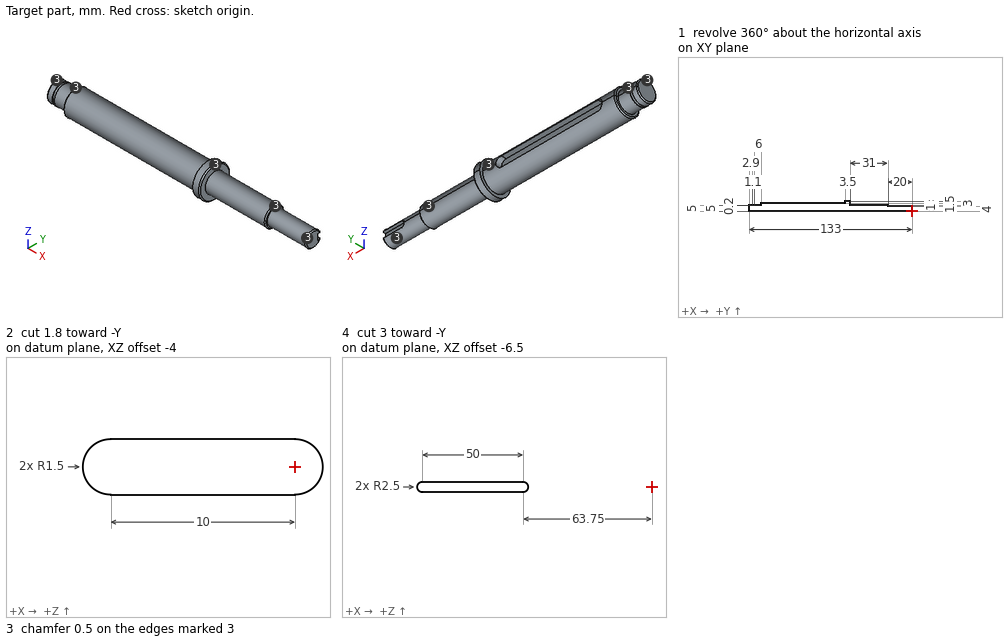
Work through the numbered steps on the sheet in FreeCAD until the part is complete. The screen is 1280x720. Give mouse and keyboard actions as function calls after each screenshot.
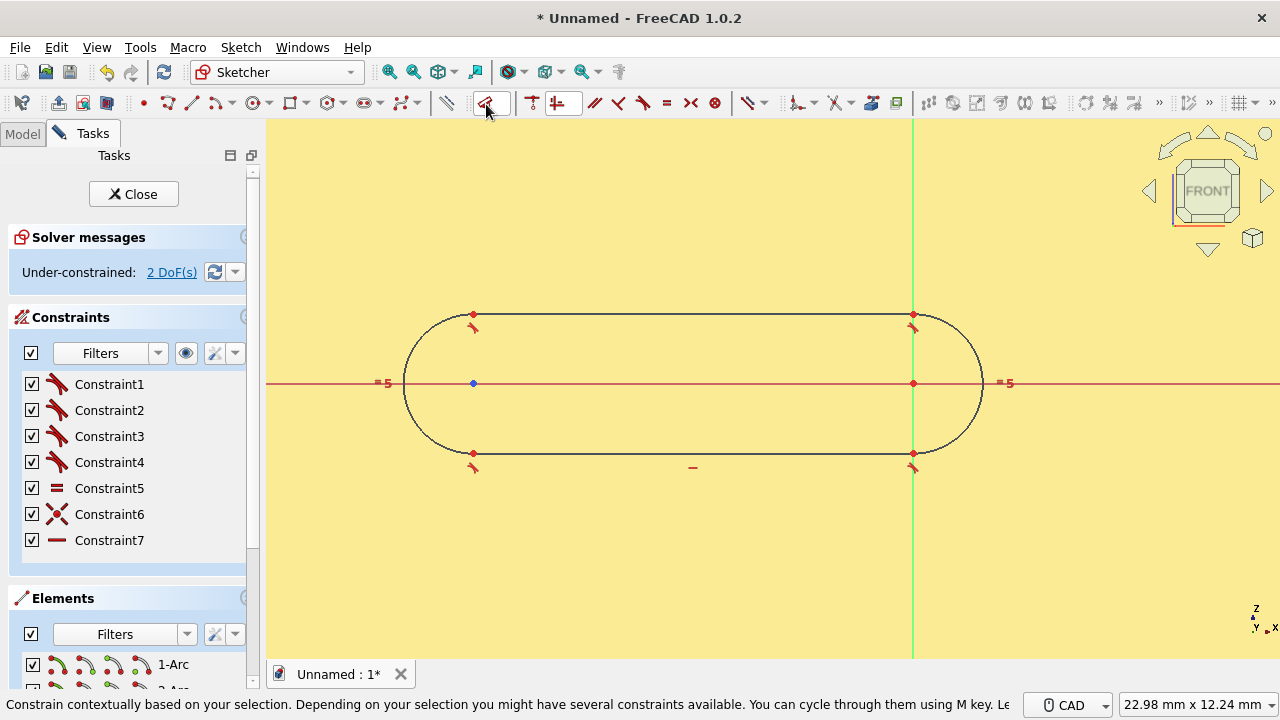
click(970, 425)
click(996, 444)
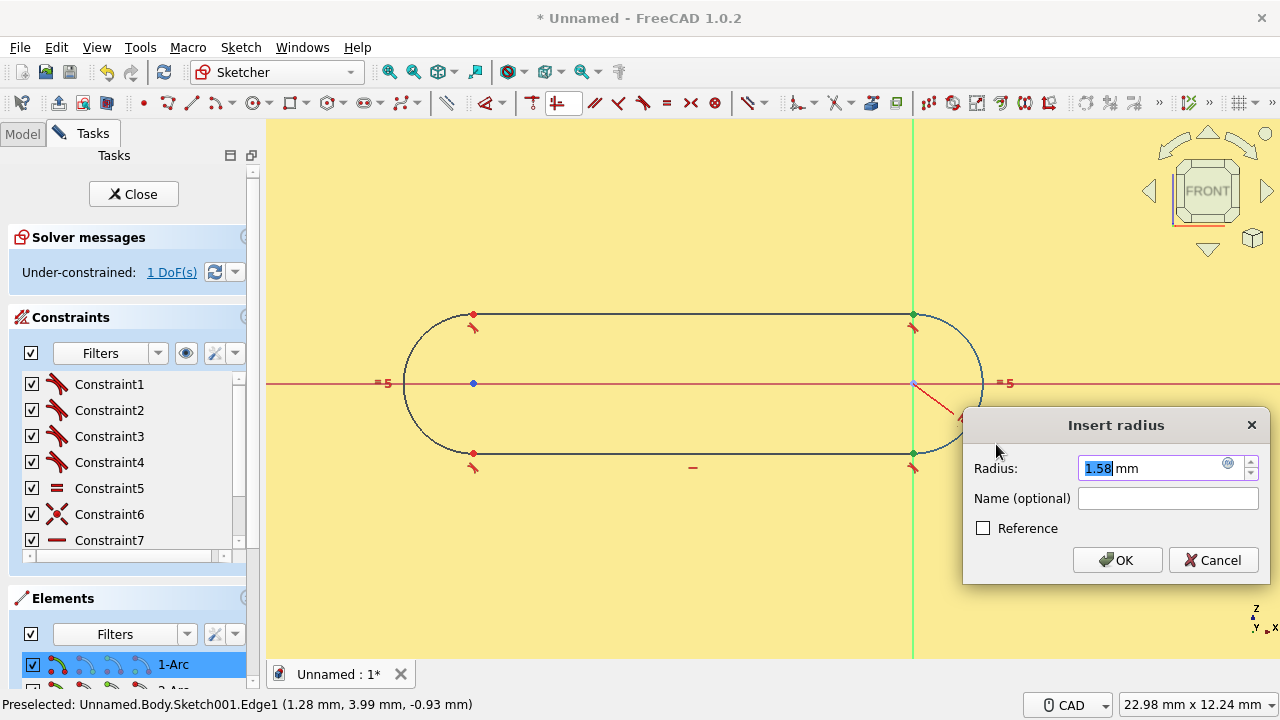
text(1.5)
key(Return)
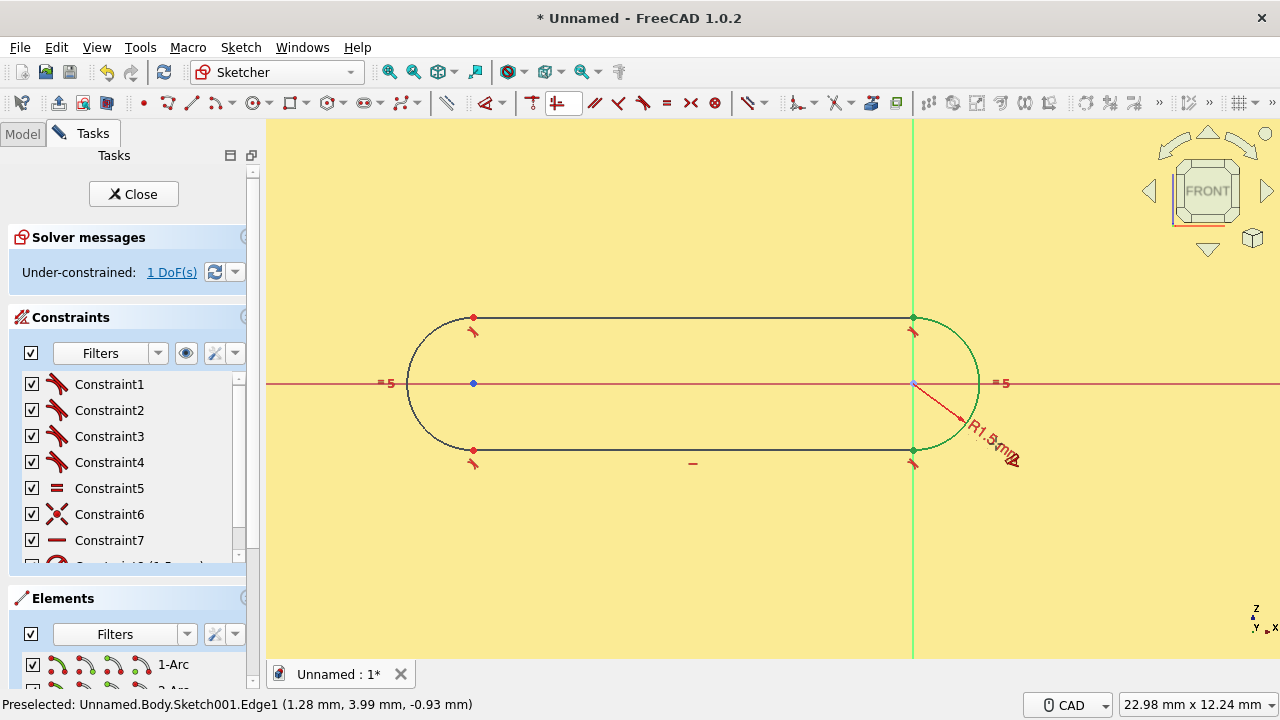
click(781, 450)
click(693, 484)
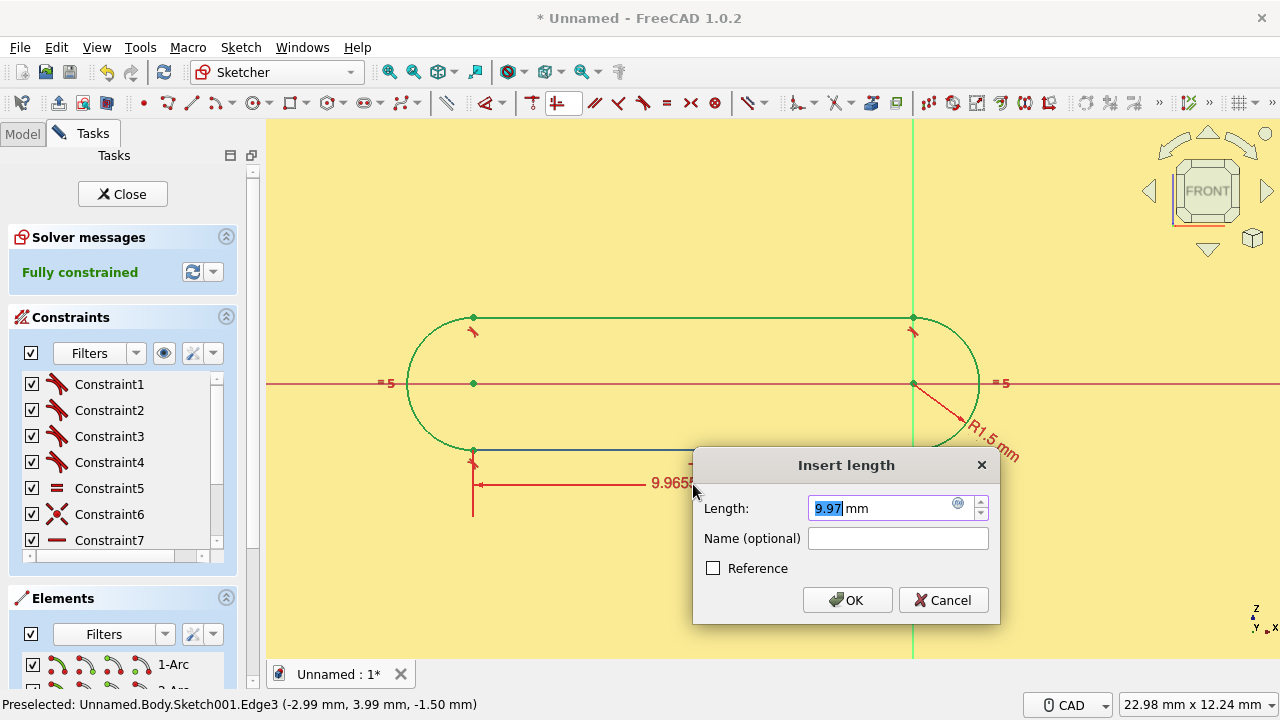
text(10)
key(Return)
key(Escape)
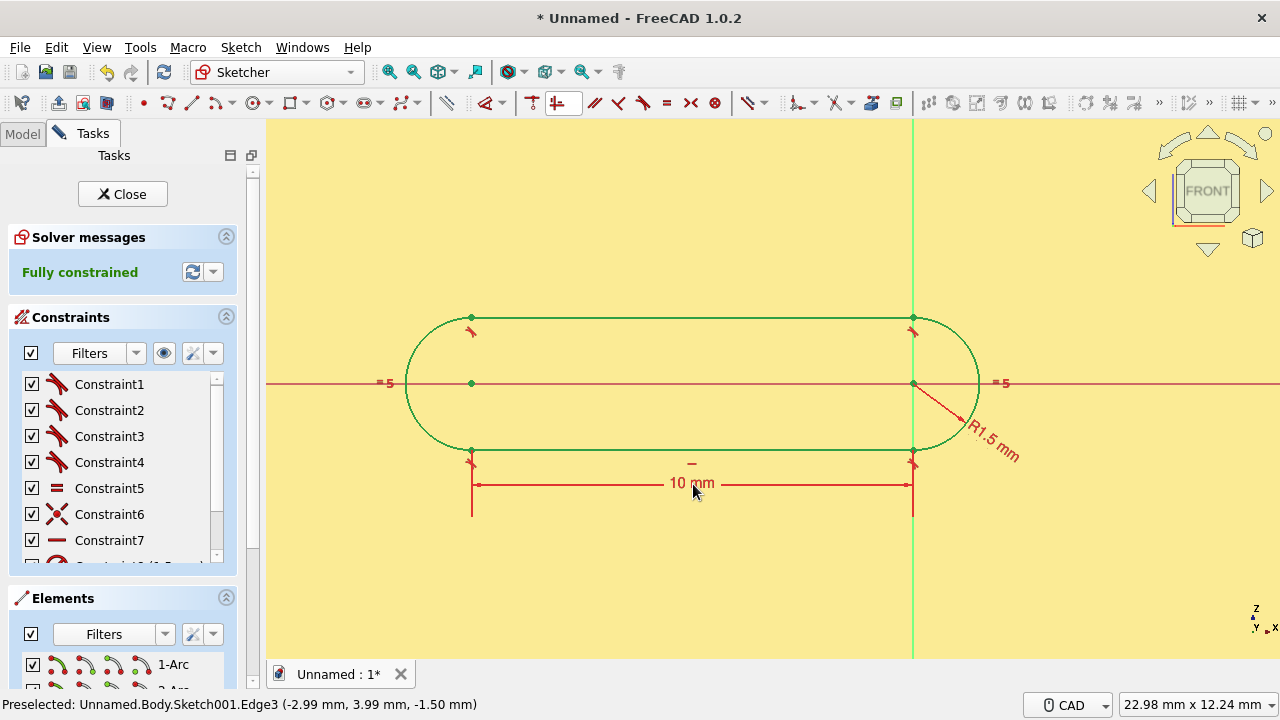
click(123, 194)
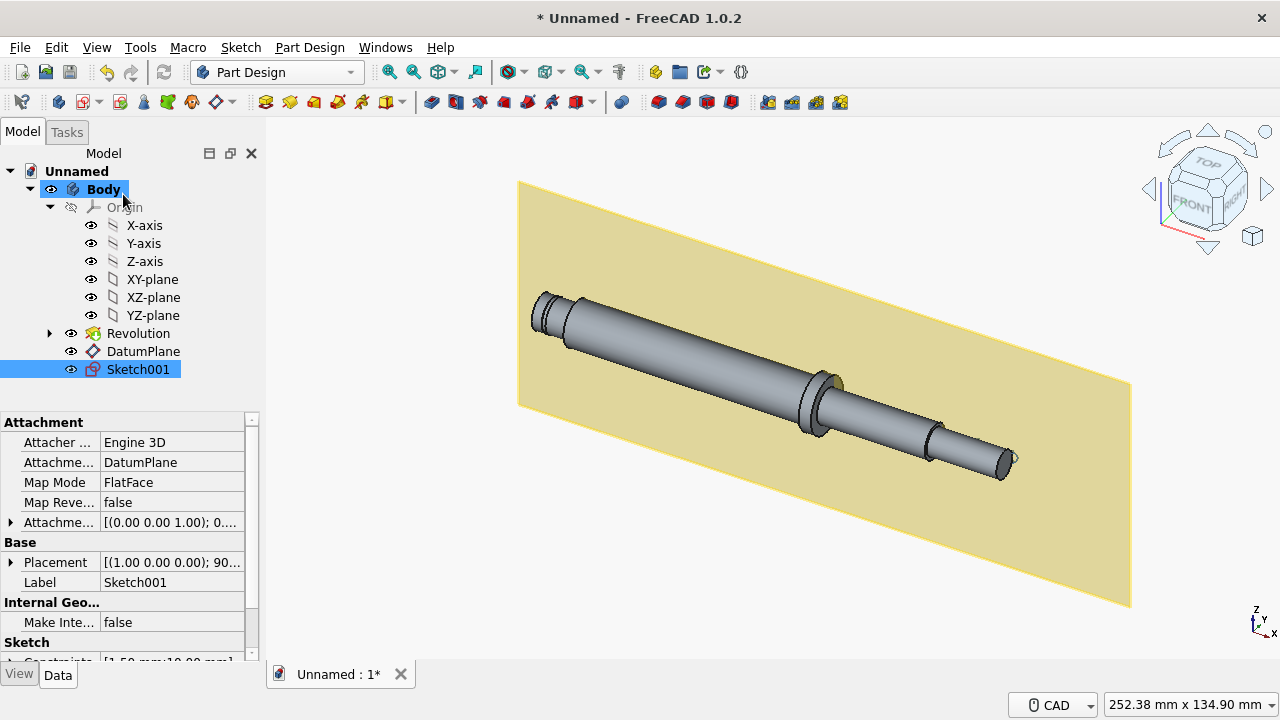
click(432, 102)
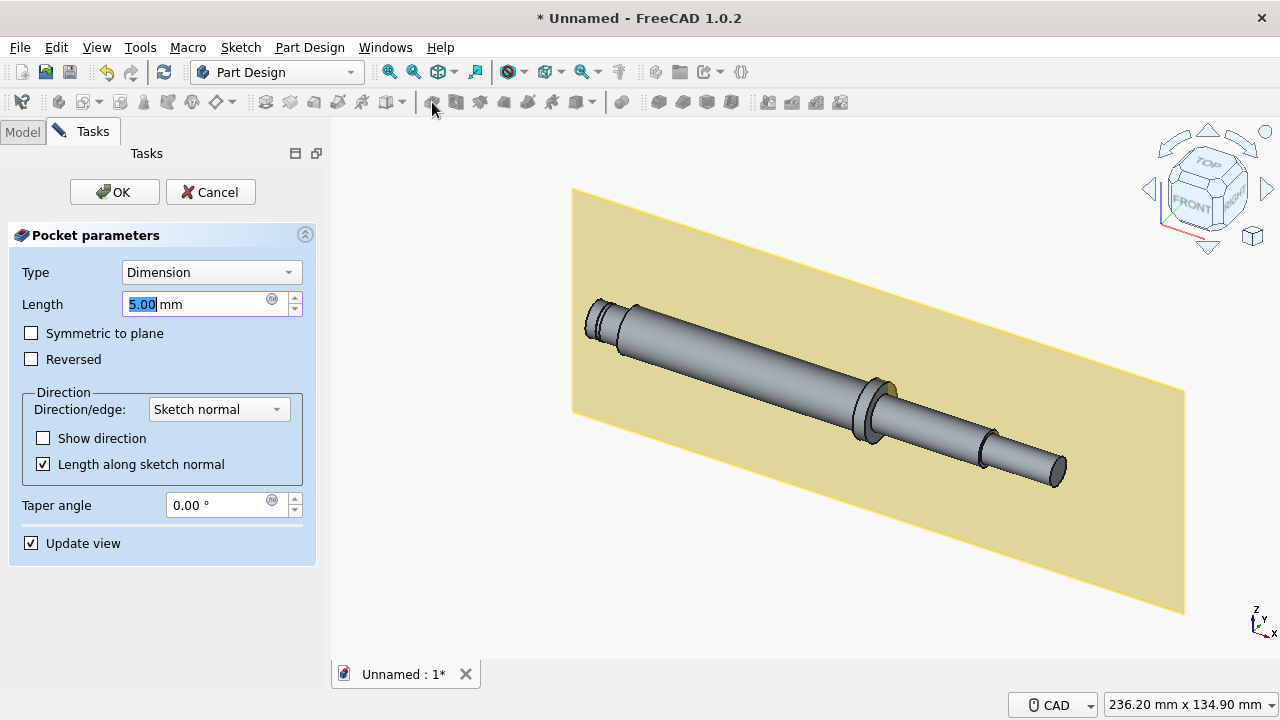
text(1.8)
key(Tab)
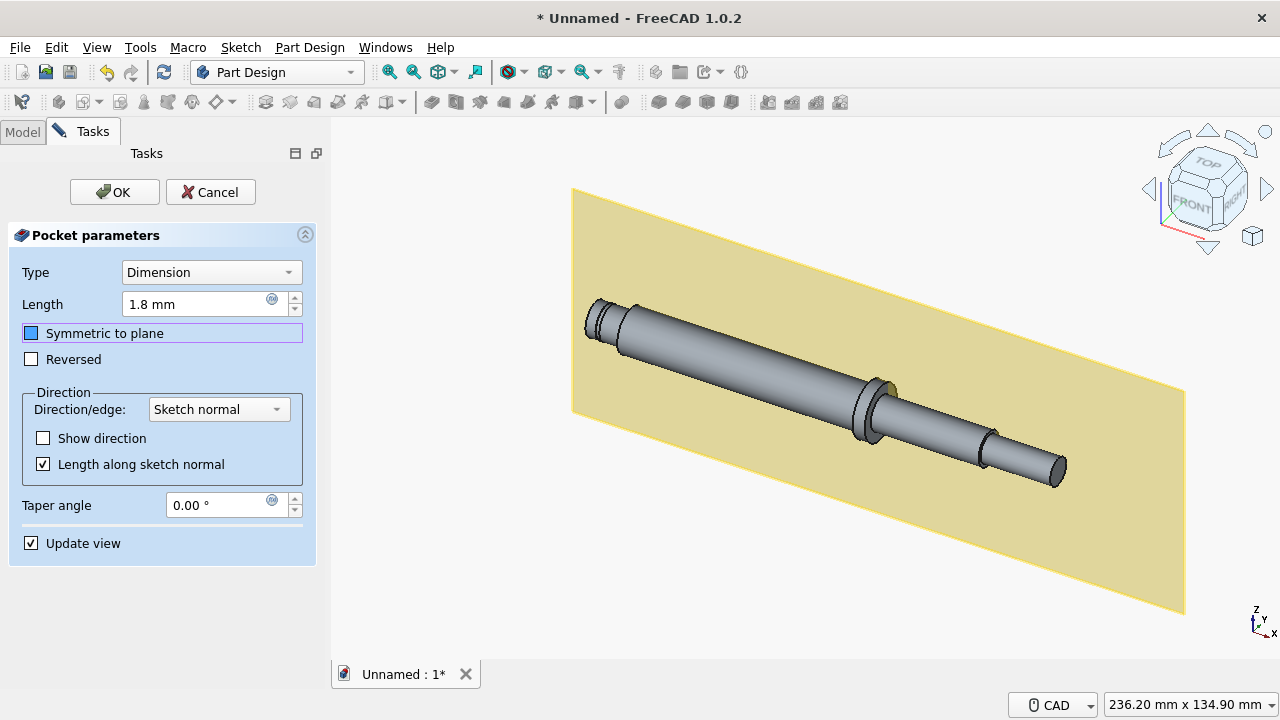
click(30, 359)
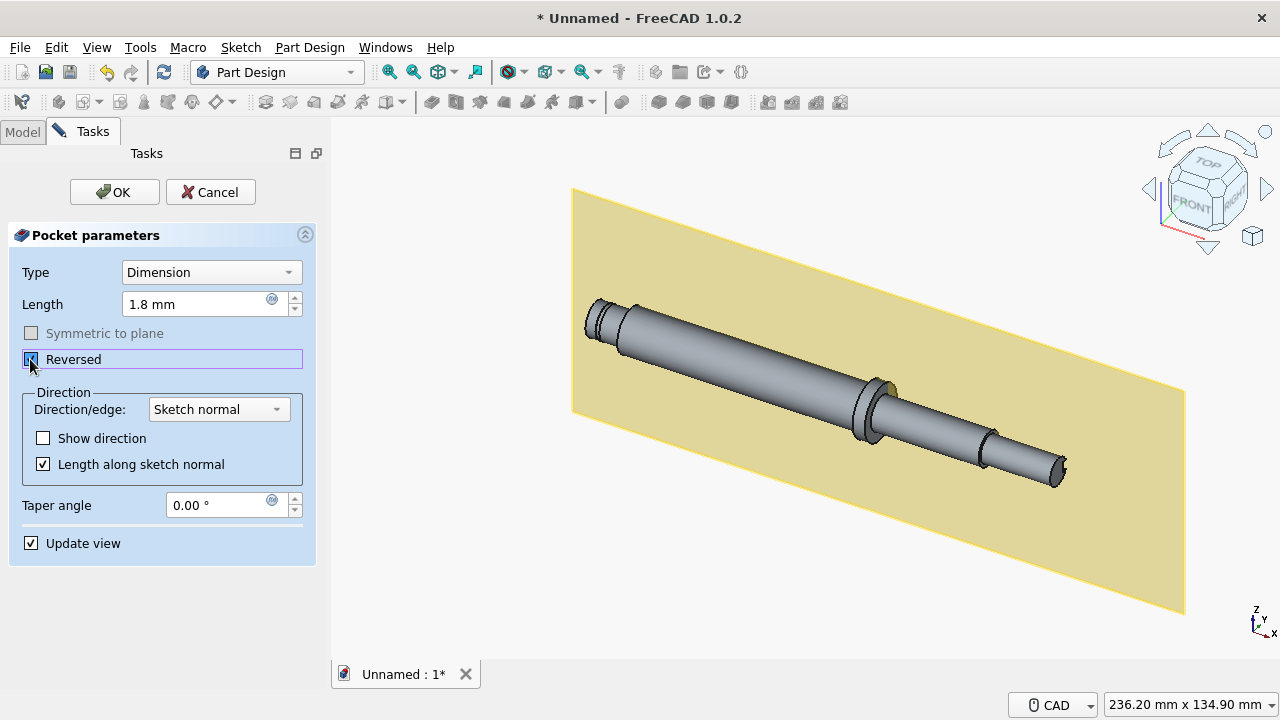
click(115, 192)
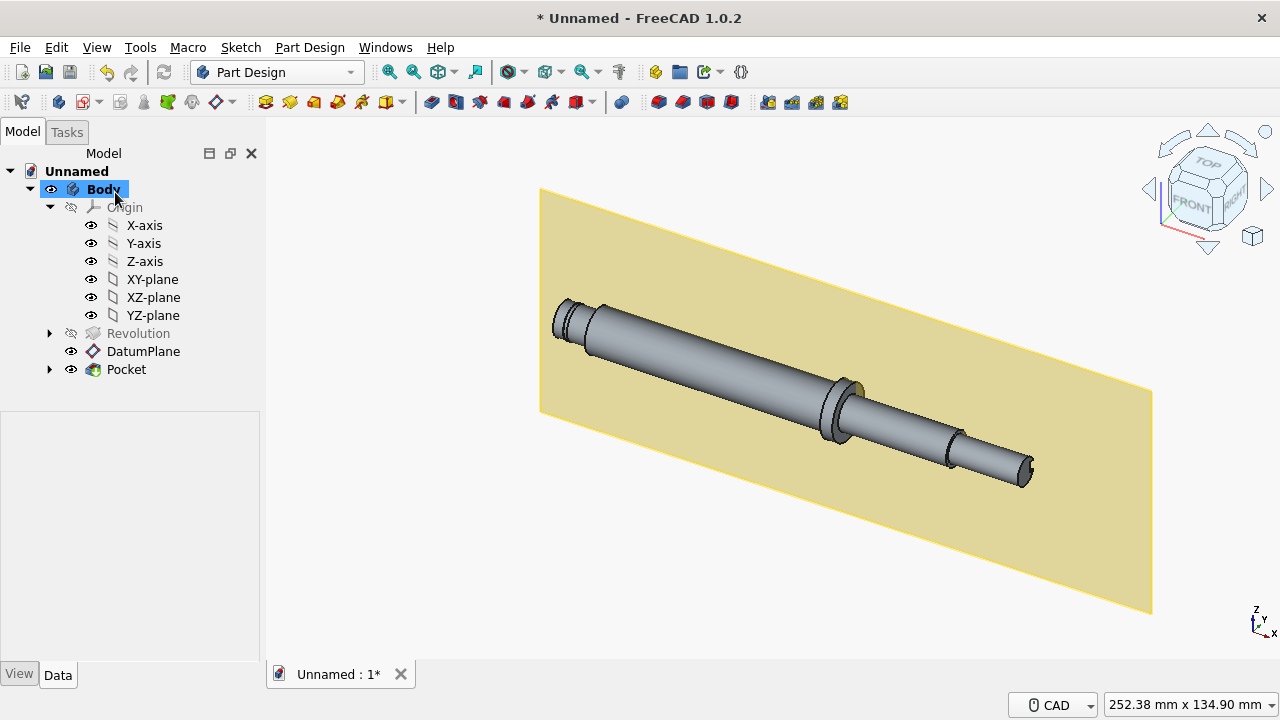
click(116, 351)
key(space)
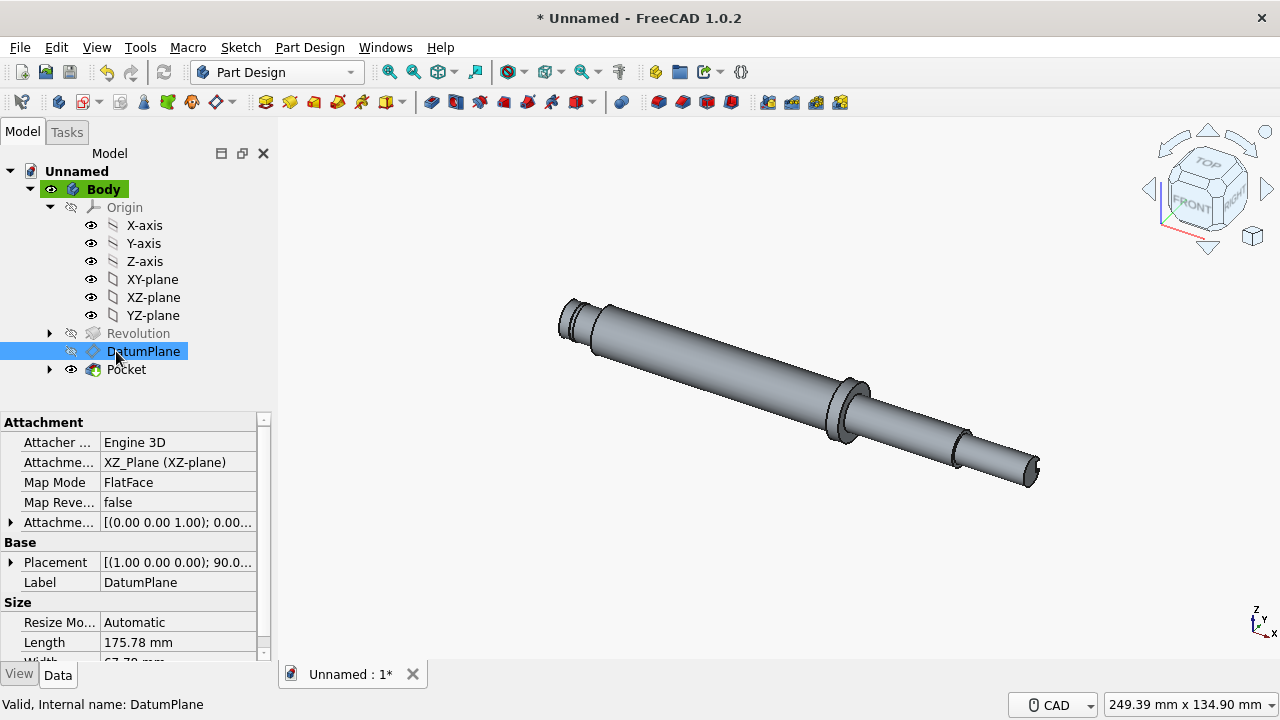
click(952, 458)